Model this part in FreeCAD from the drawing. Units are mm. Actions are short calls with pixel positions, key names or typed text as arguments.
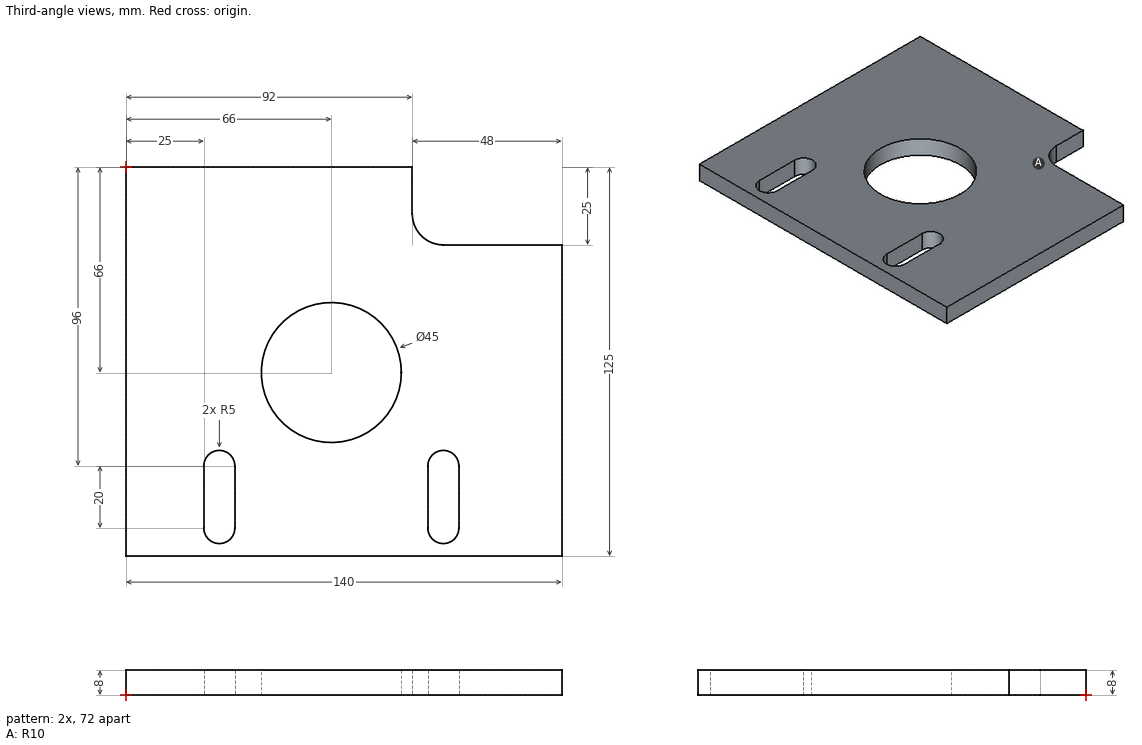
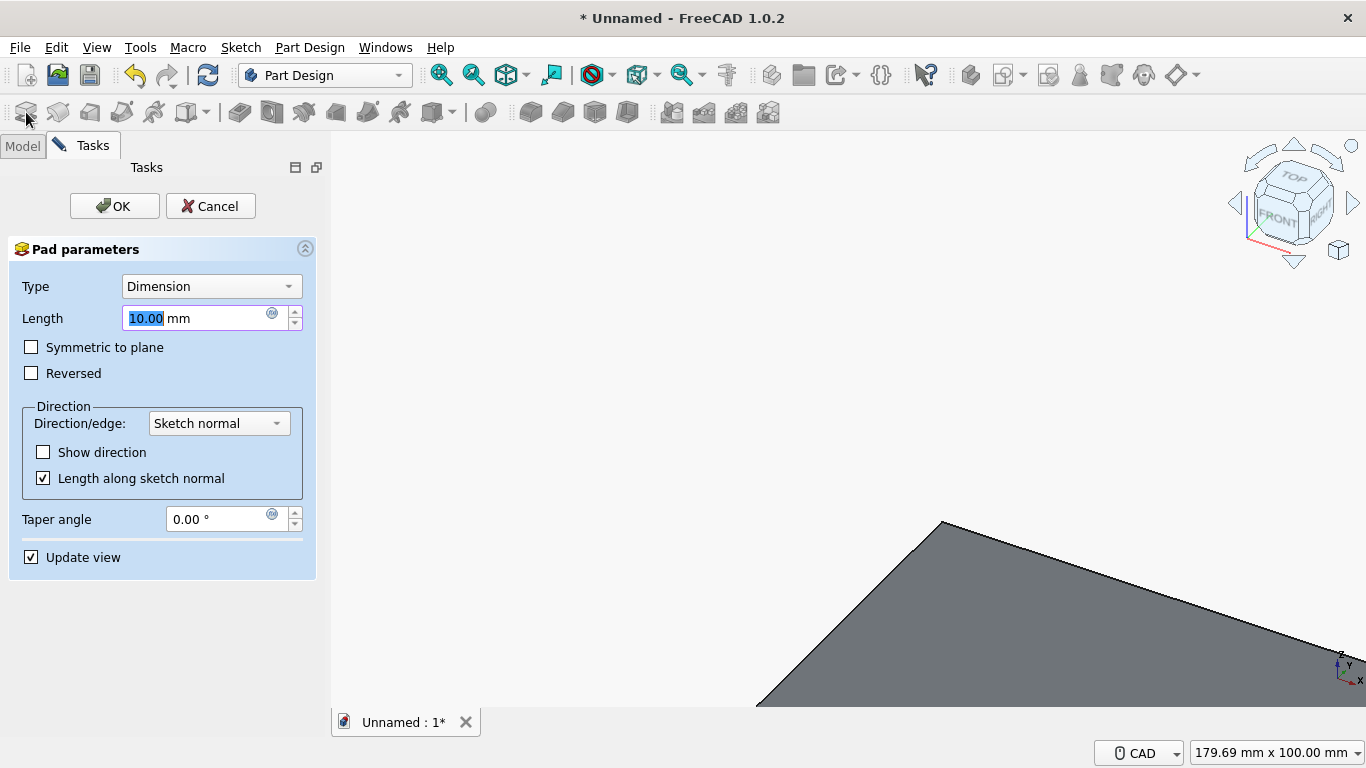
text(8)
key(Tab)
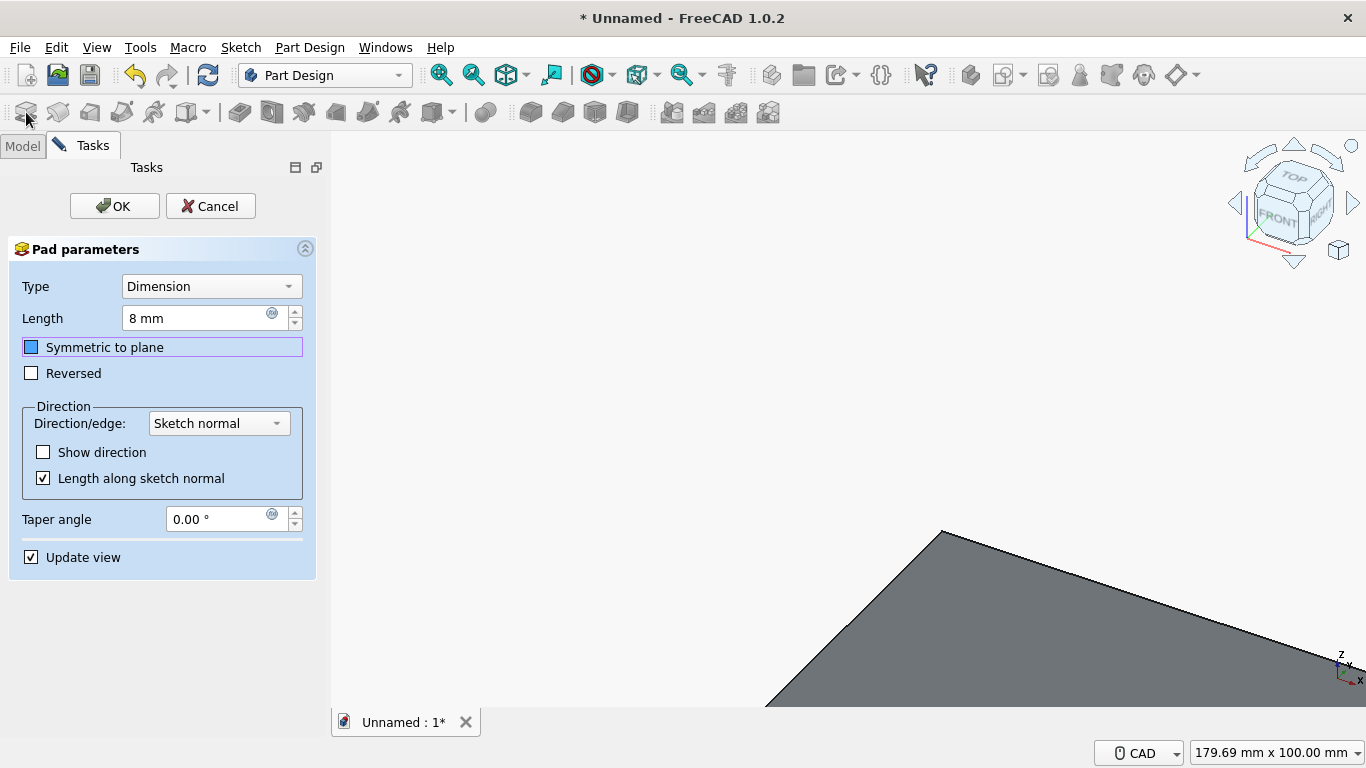
click(115, 206)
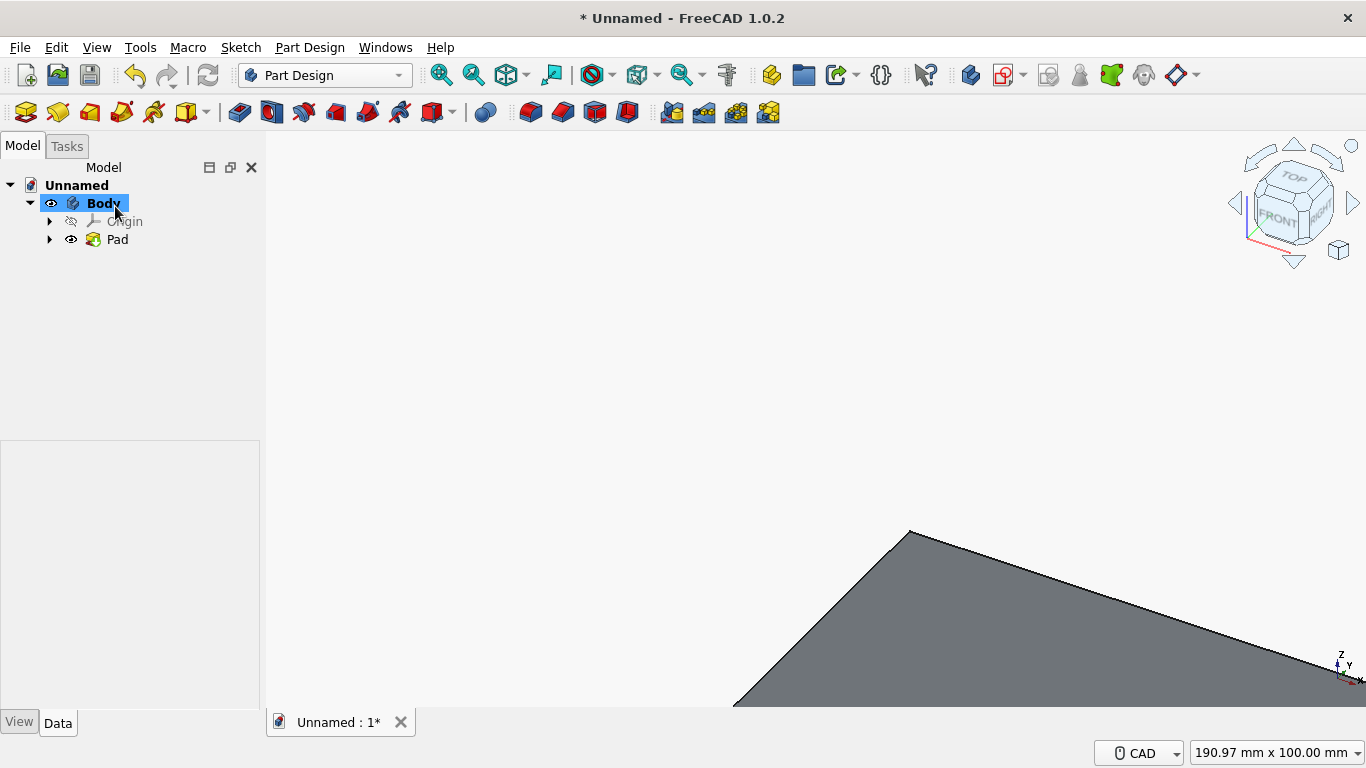
key(v)
key(f)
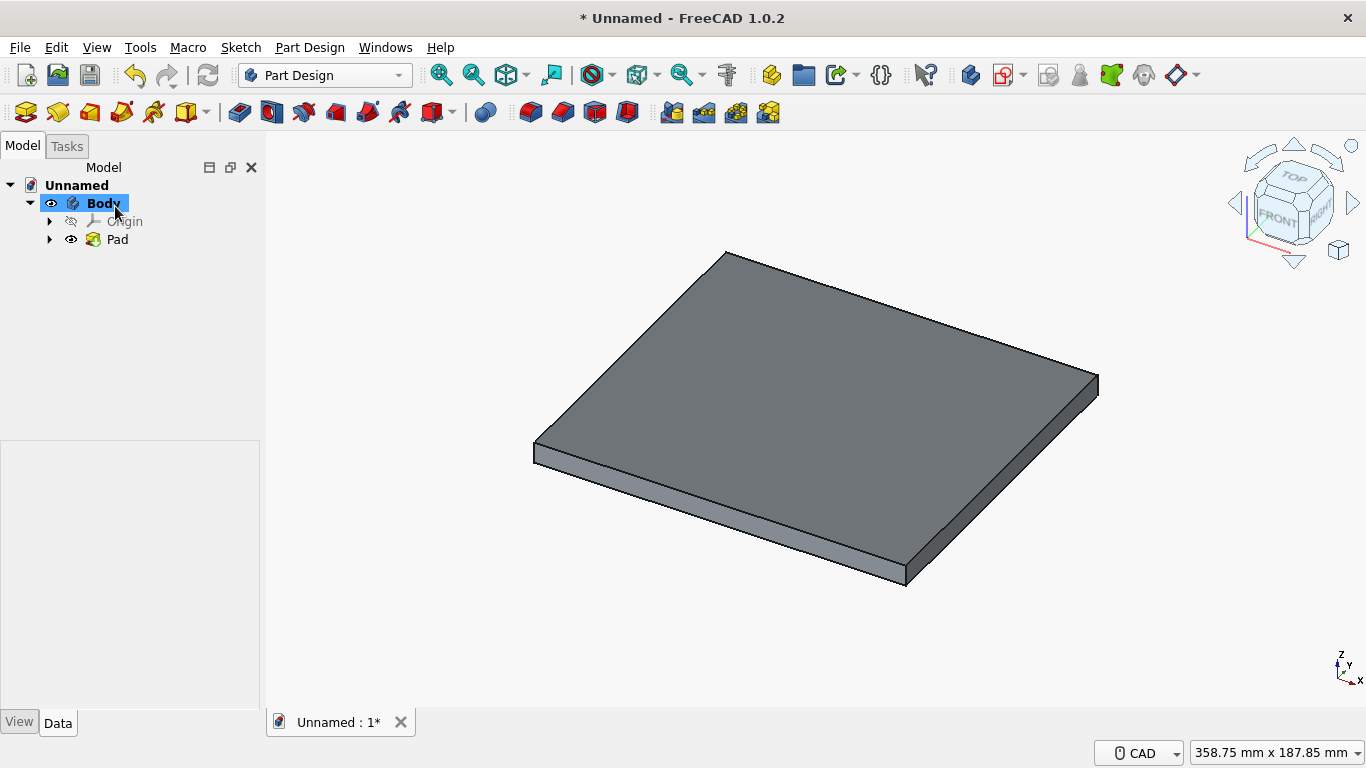
click(816, 408)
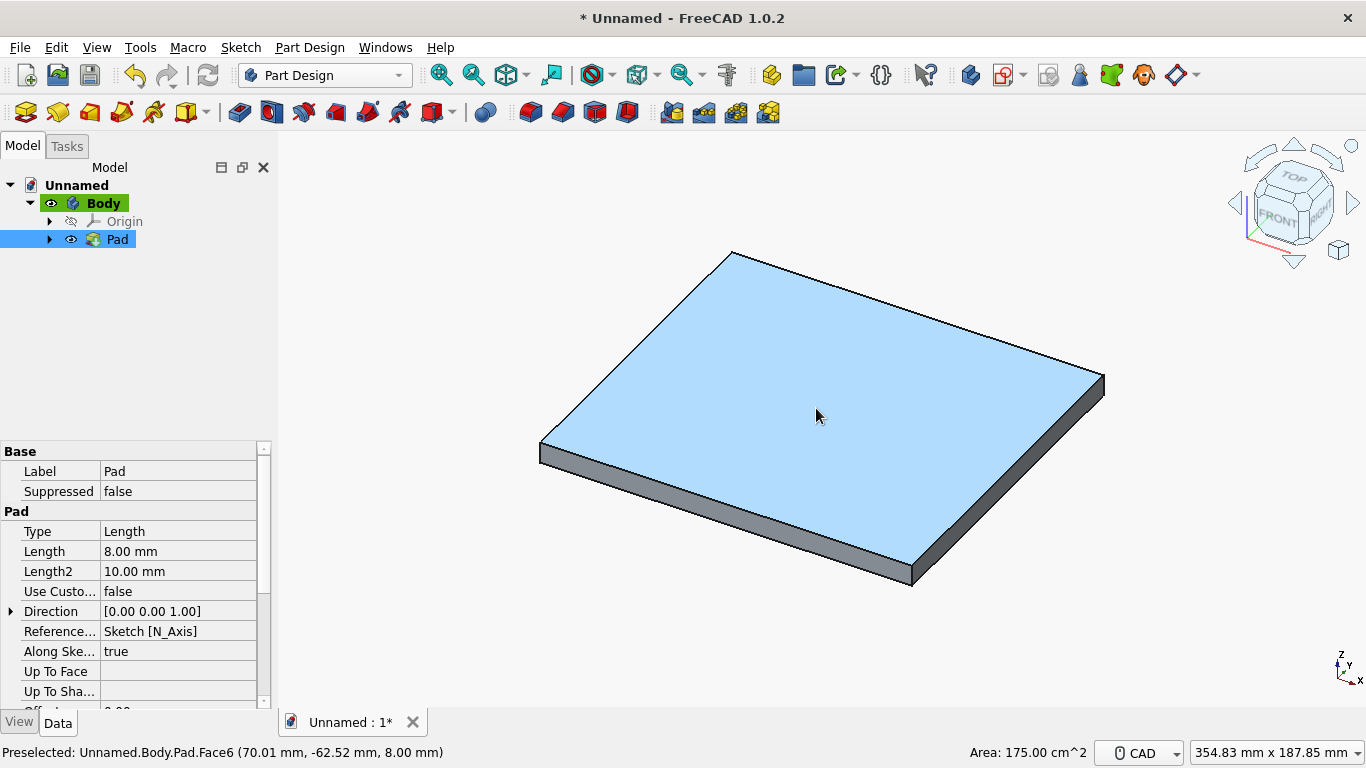
click(1004, 76)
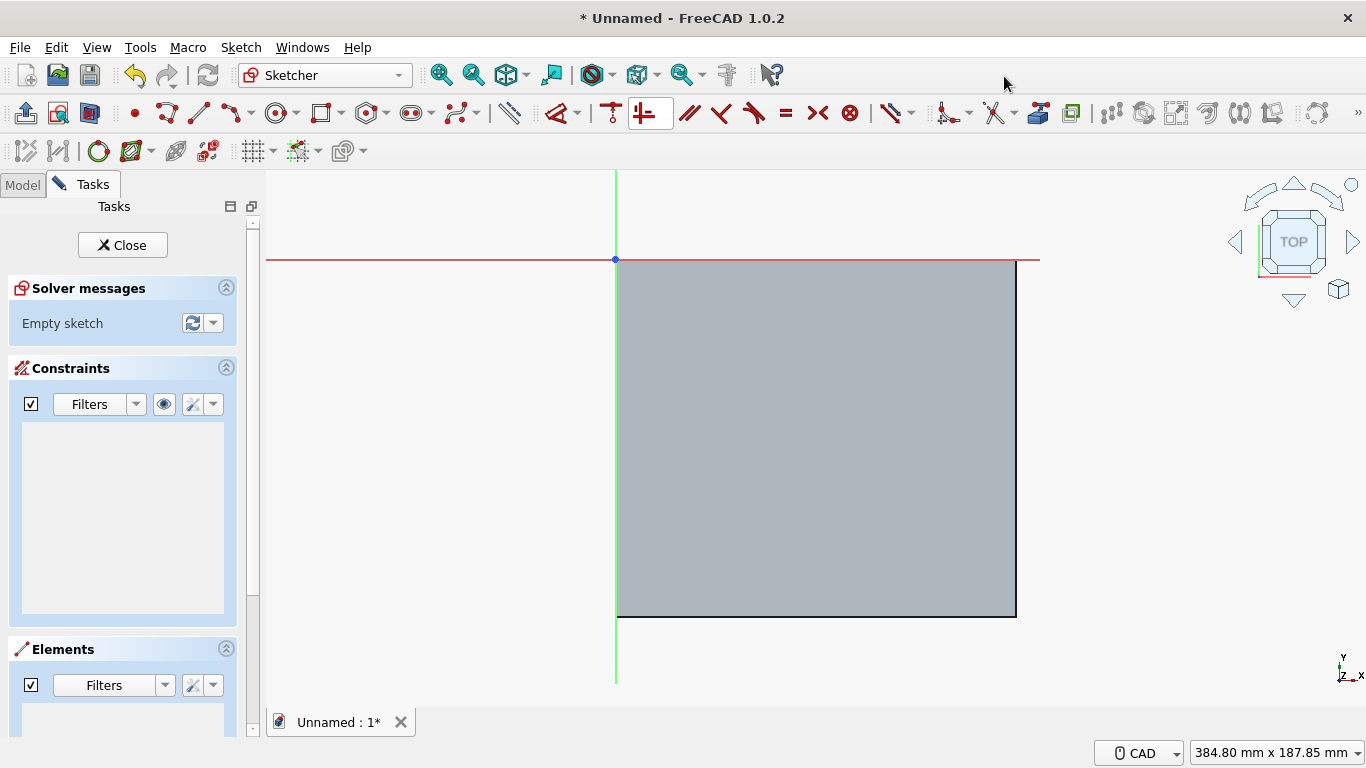
click(276, 114)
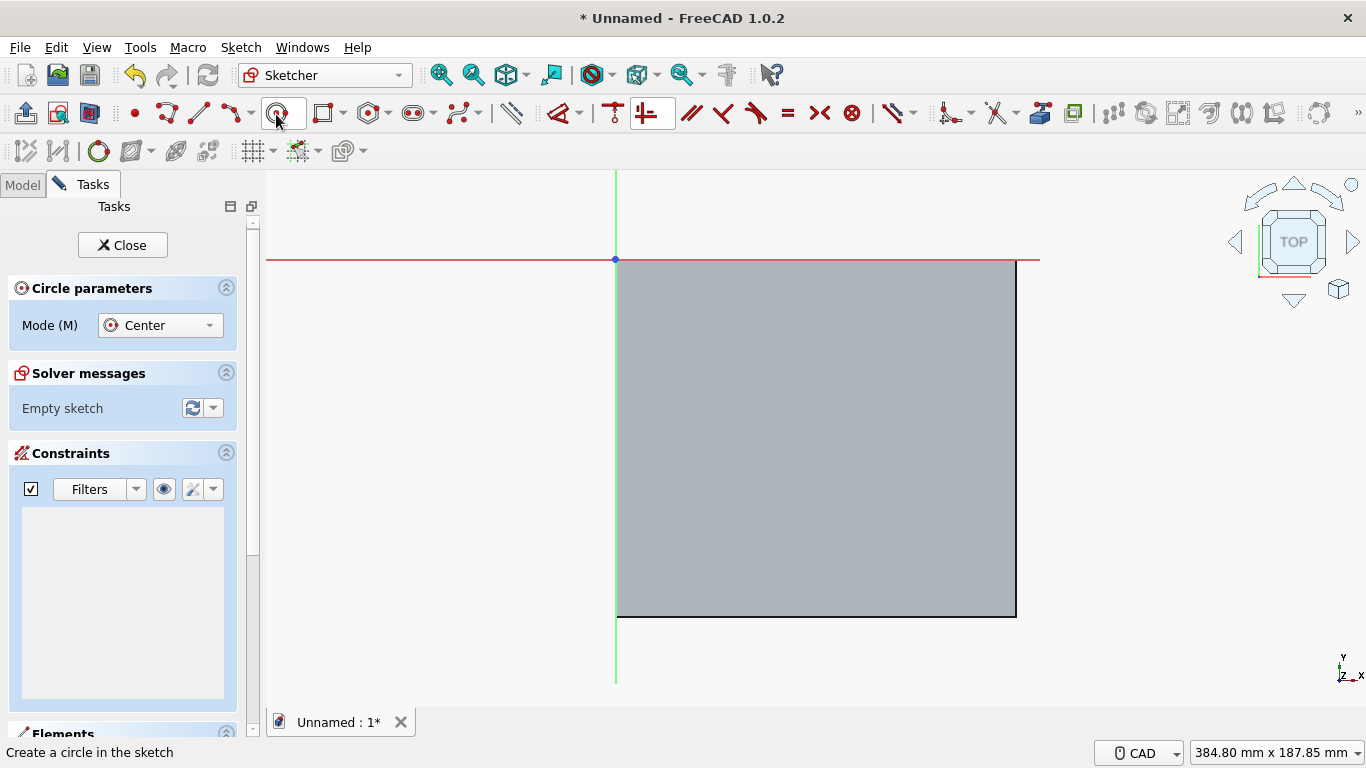
click(805, 449)
move(850, 403)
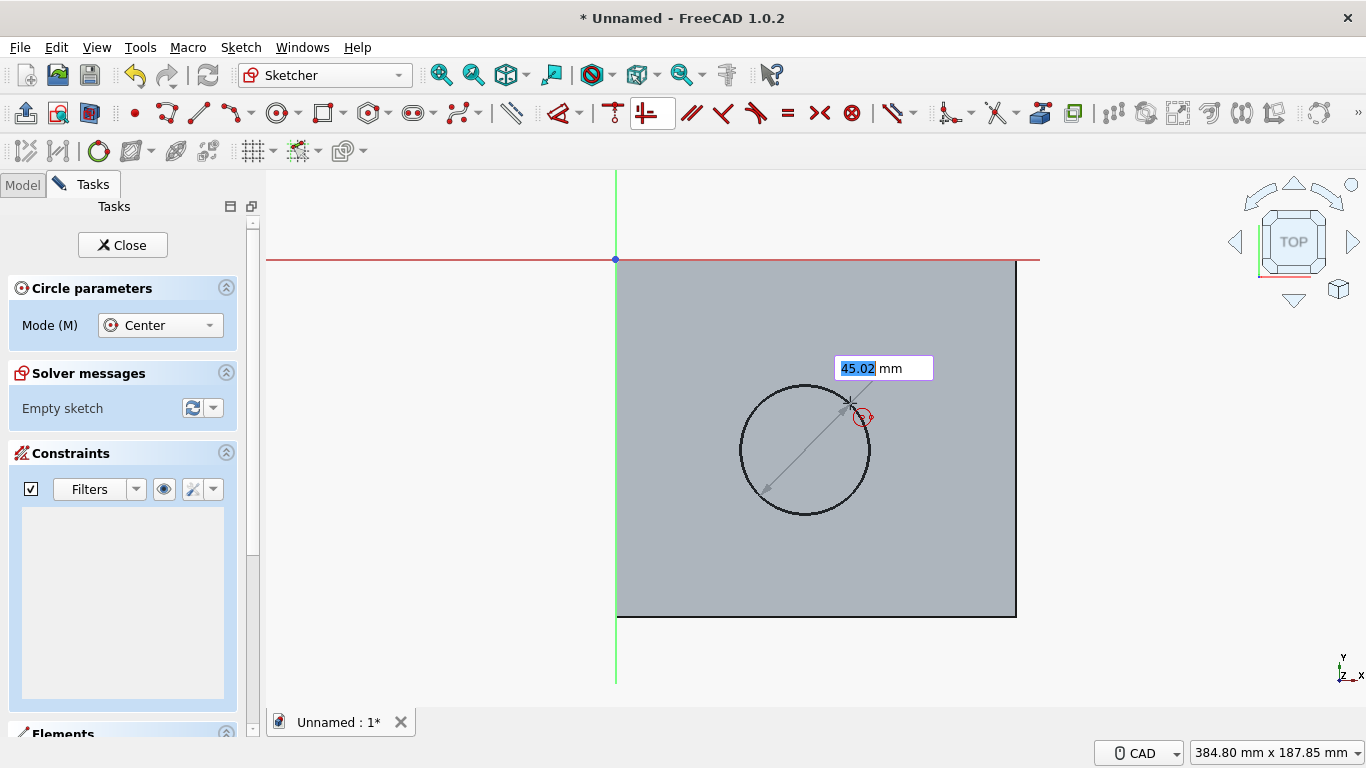
text(45)
key(Return)
key(Escape)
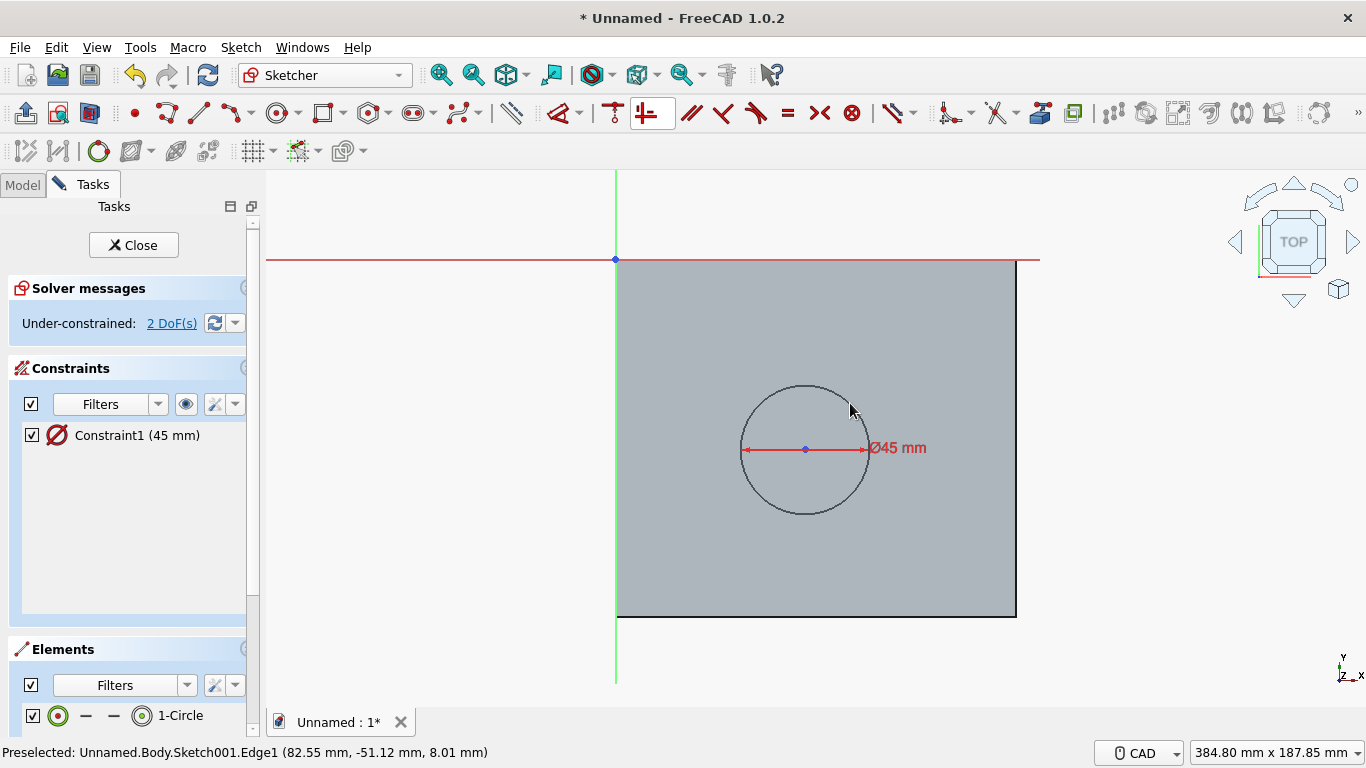
click(805, 450)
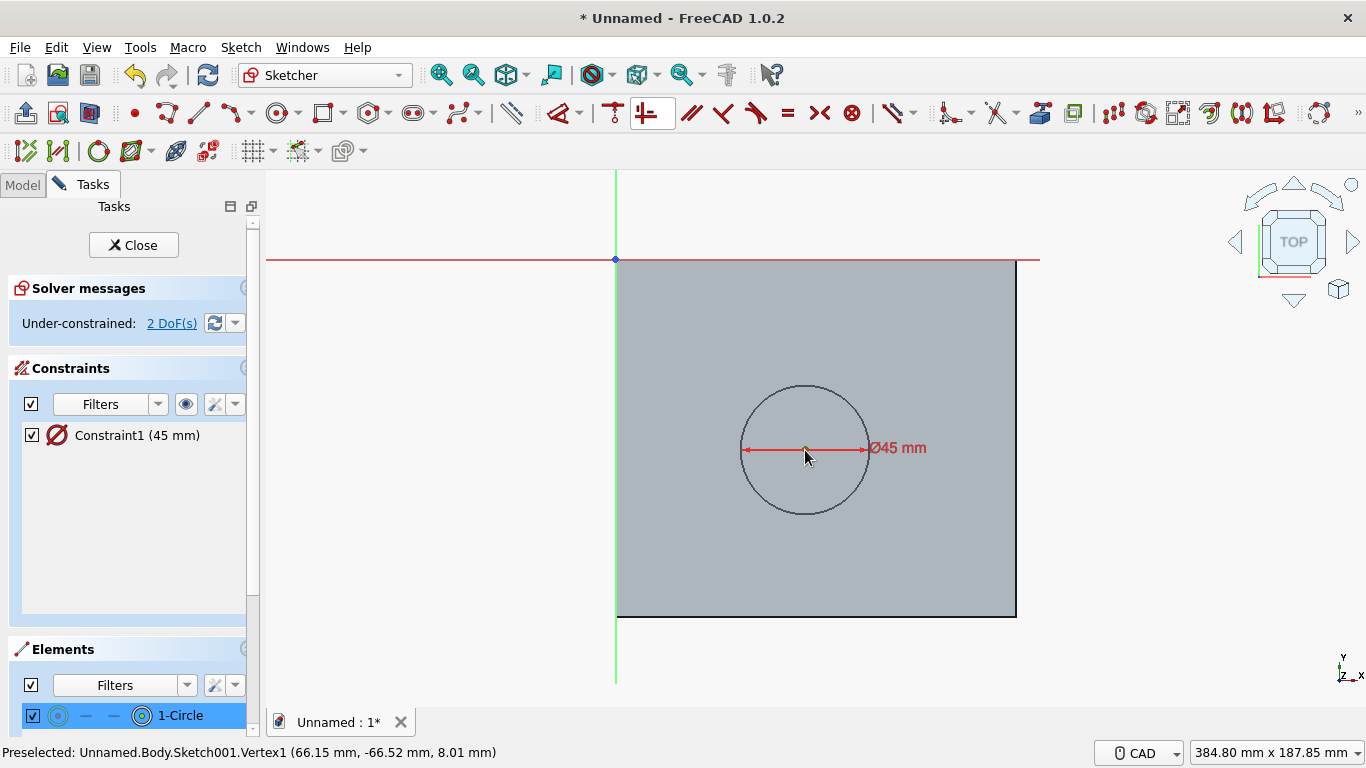
key(l)